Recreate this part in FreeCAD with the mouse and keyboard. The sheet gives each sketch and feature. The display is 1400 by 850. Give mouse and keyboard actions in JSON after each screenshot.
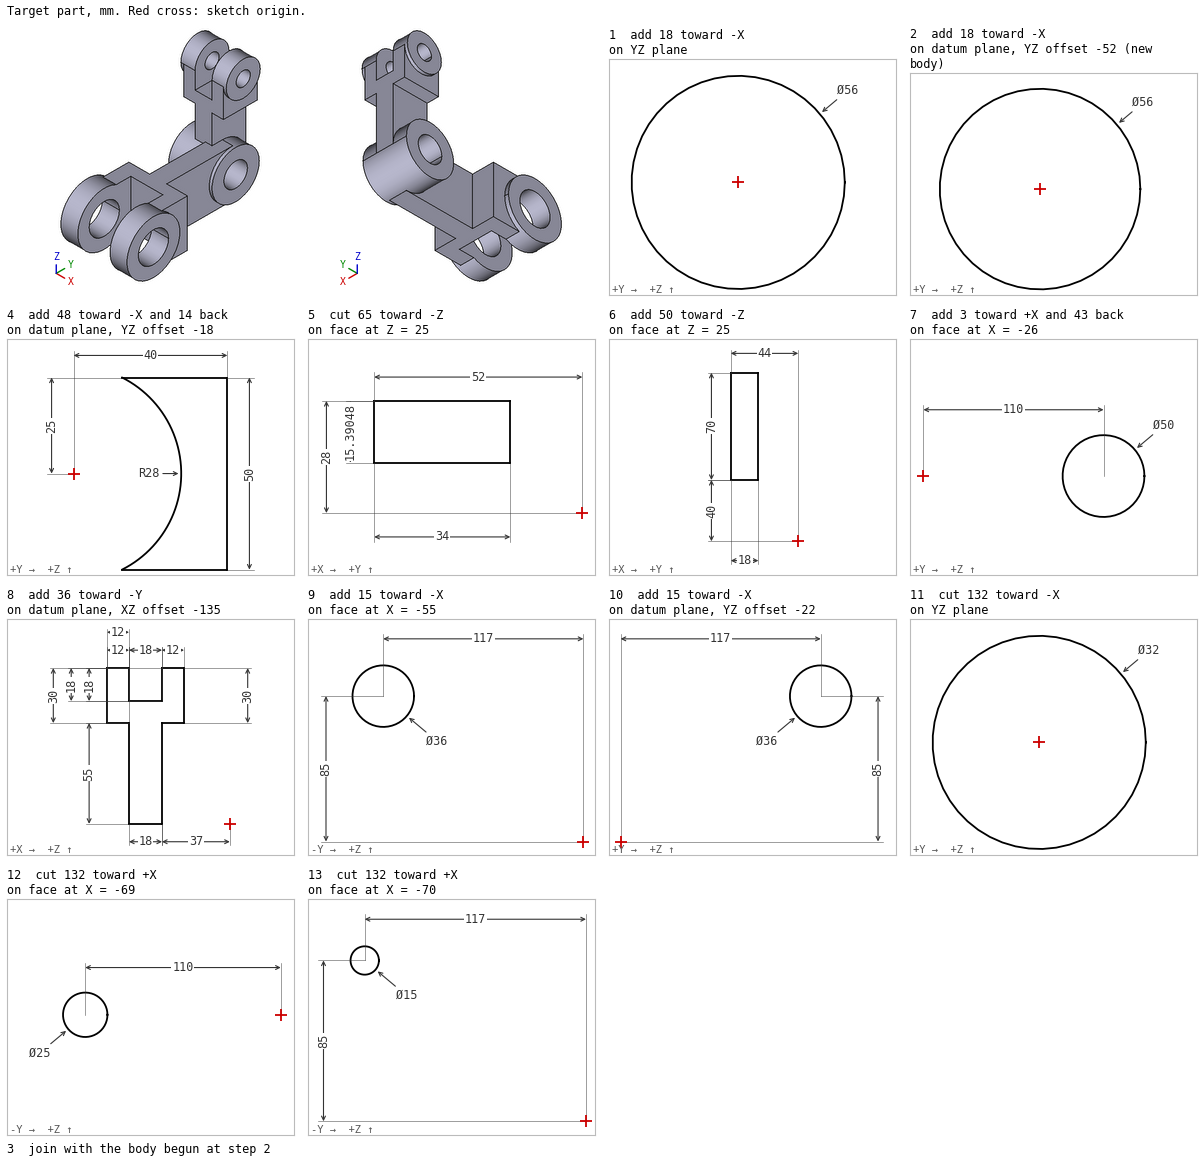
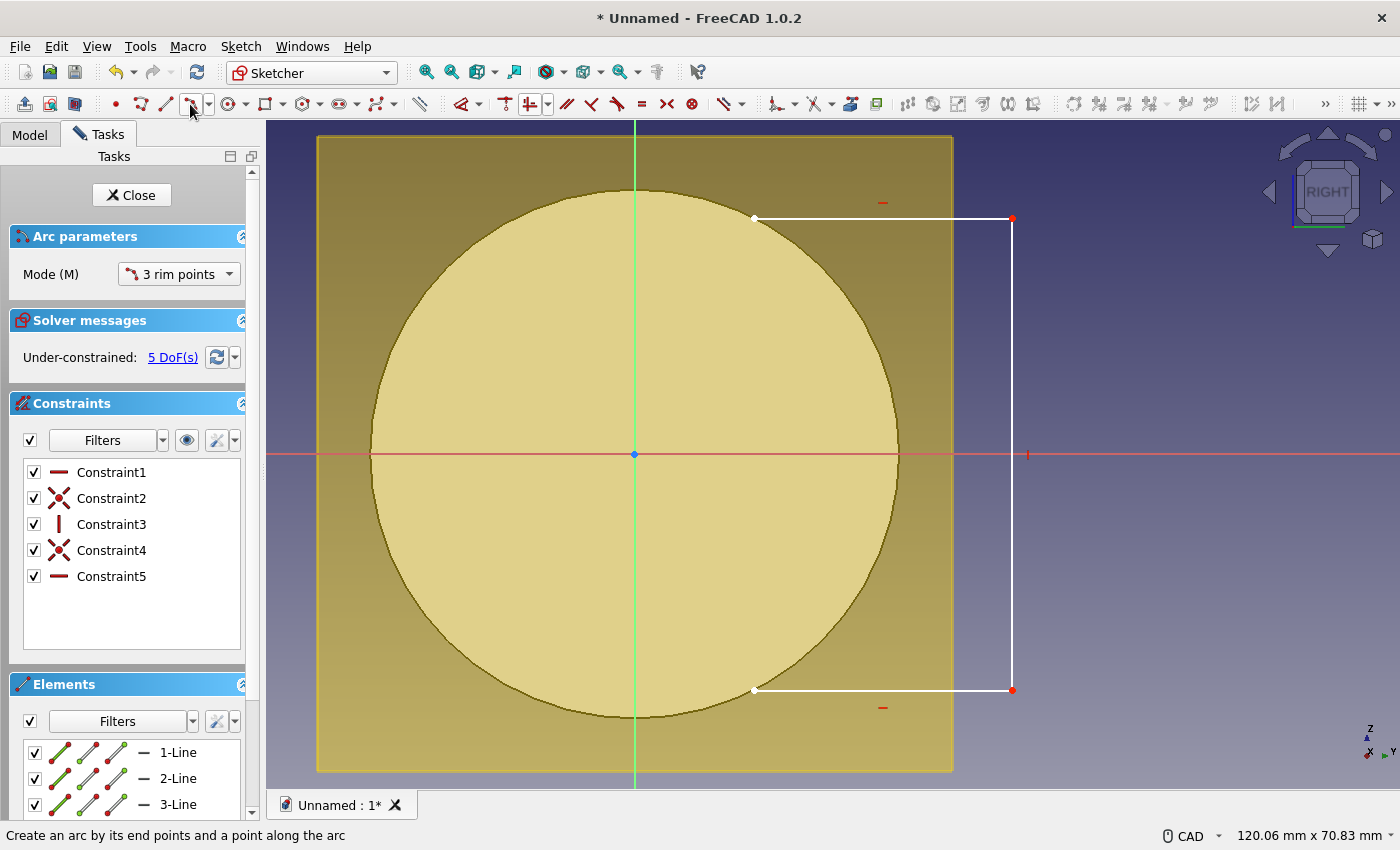
{"action": "left_click", "coordinate": [754, 691]}
{"action": "left_click", "coordinate": [754, 219]}
{"action": "left_click", "coordinate": [893, 512]}
{"action": "key", "text": "Escape"}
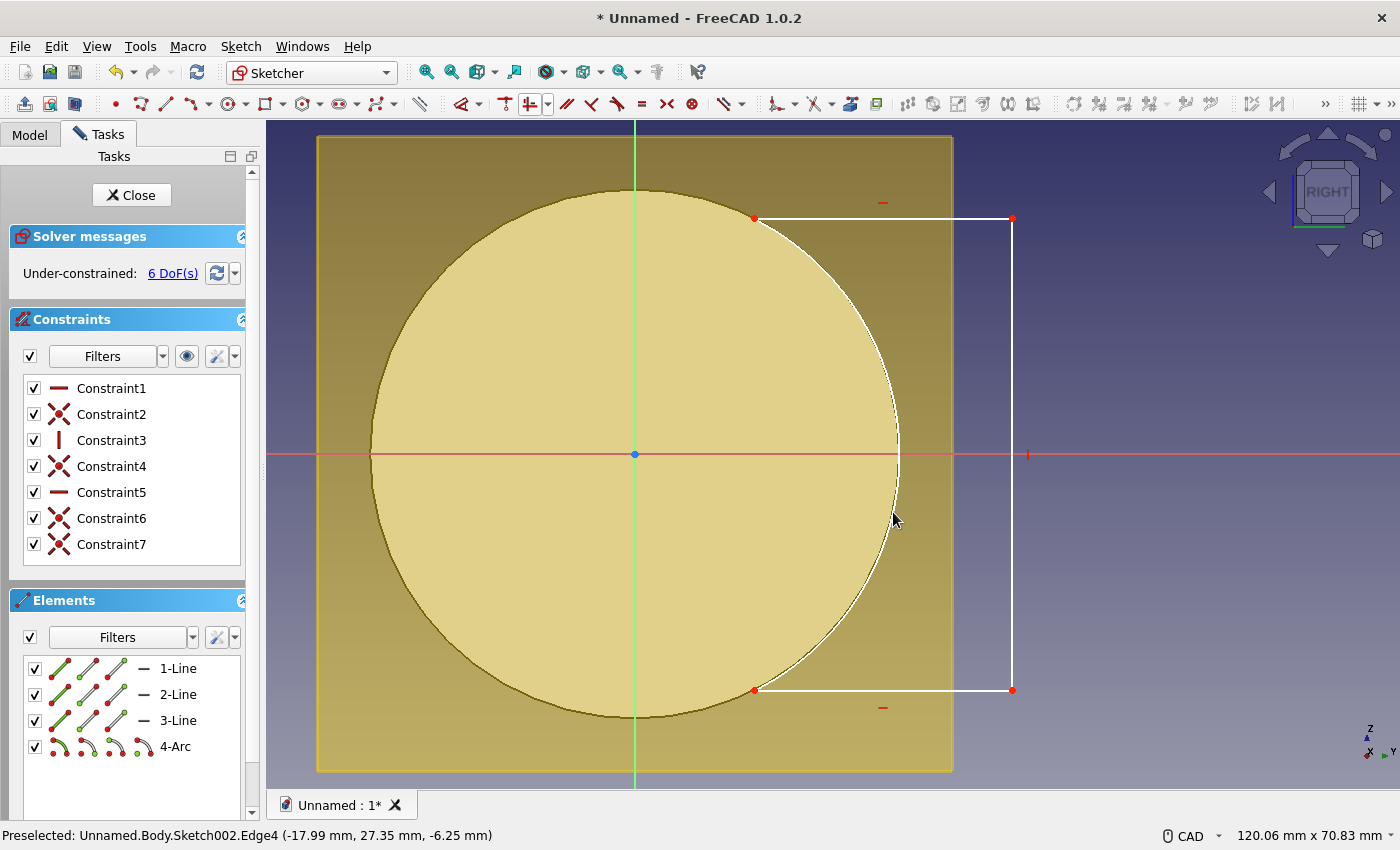
{"action": "left_click_drag", "start_coordinate": [625, 444], "coordinate": [645, 465]}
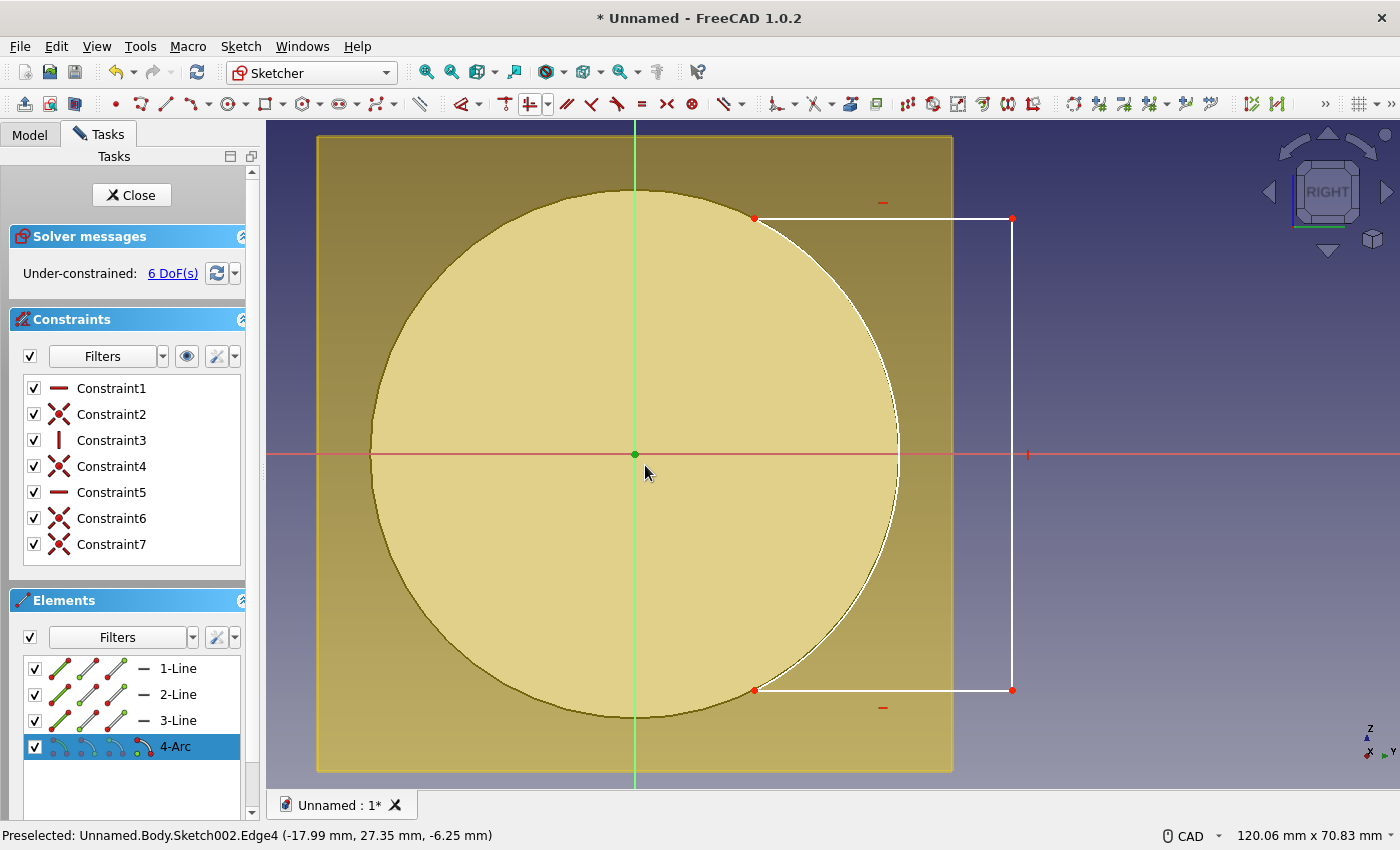
{"action": "key", "text": "c"}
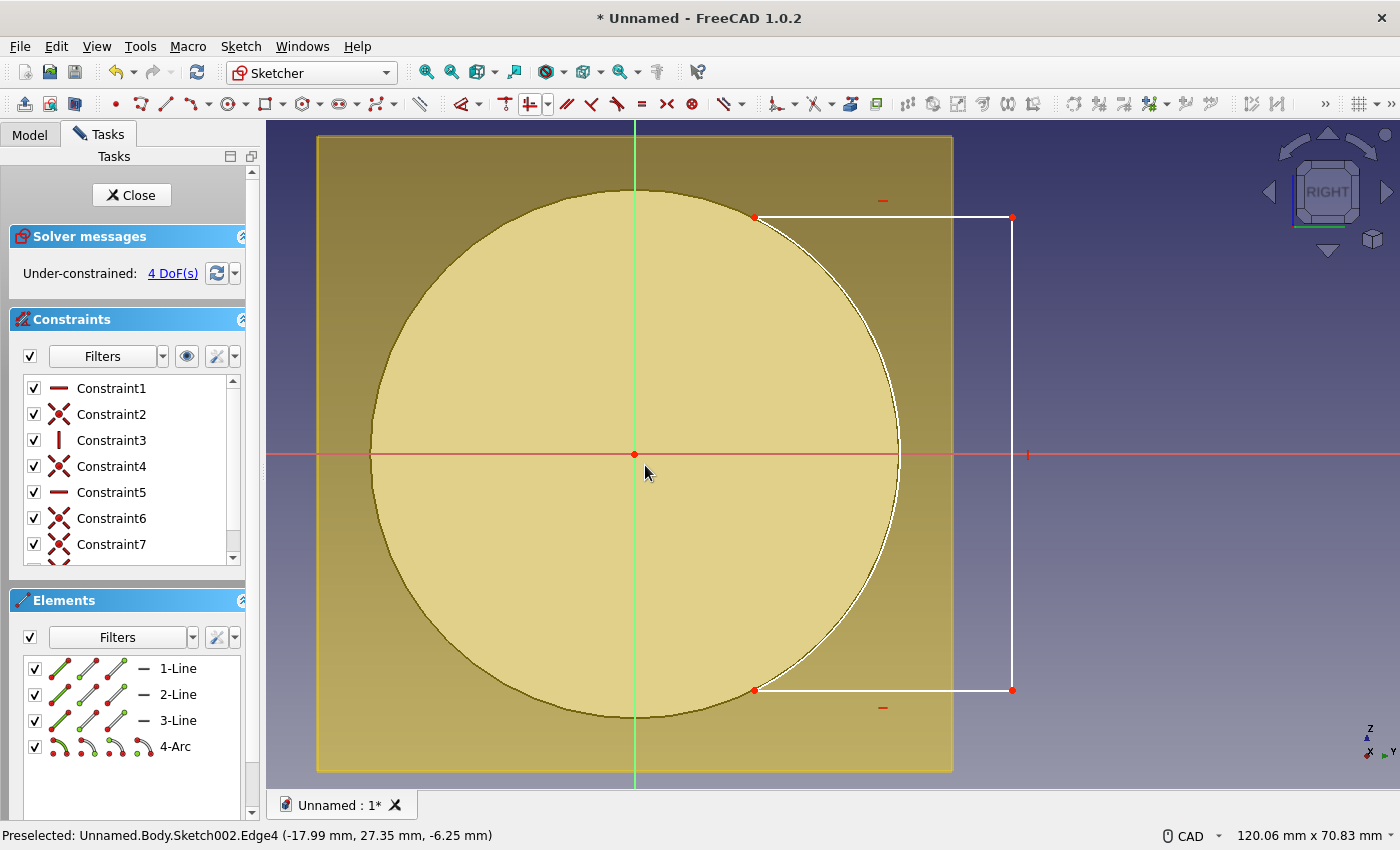
{"action": "left_click", "coordinate": [875, 567]}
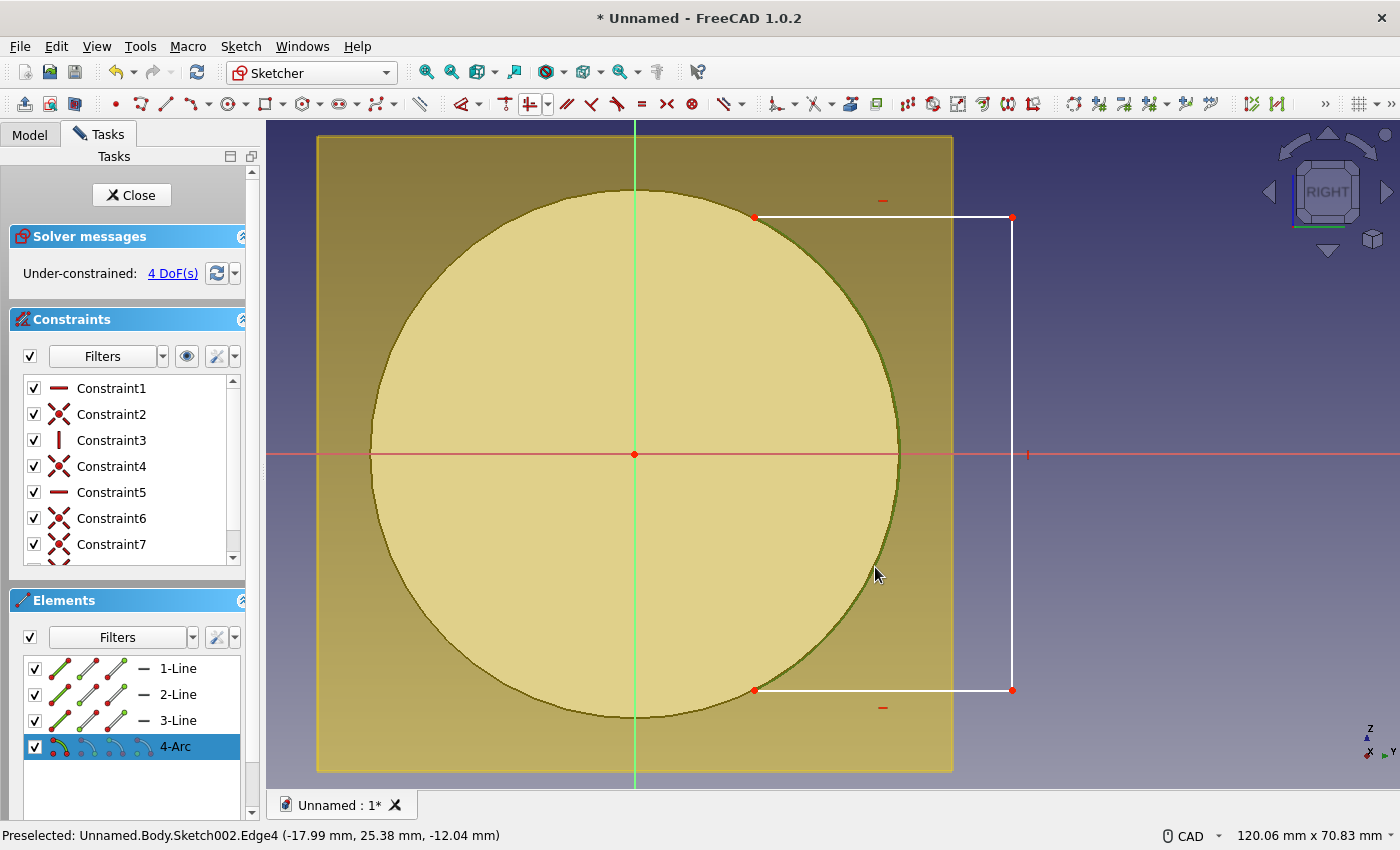
{"action": "key", "text": "k r"}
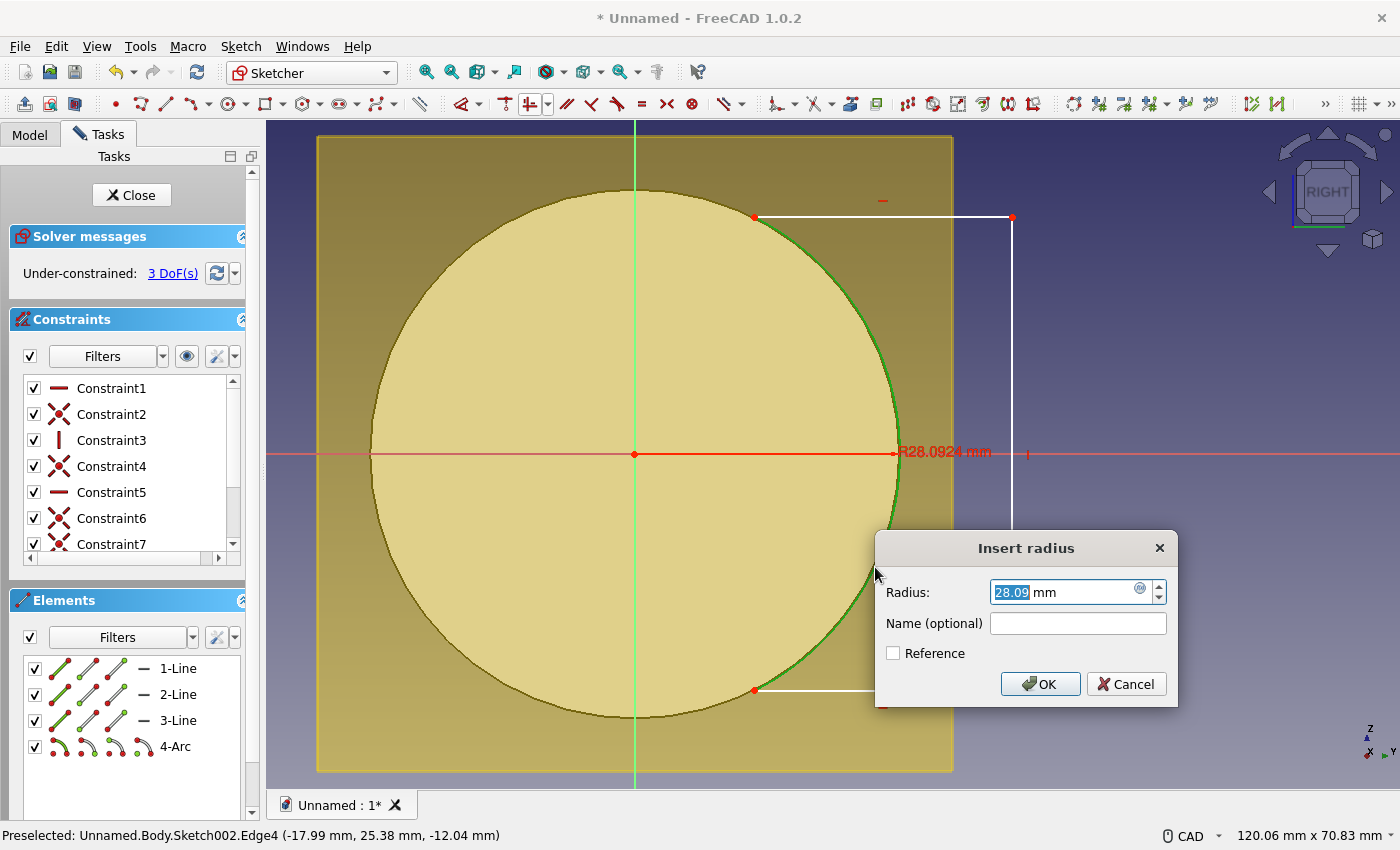
{"action": "type", "text": "28"}
{"action": "key", "text": "Return"}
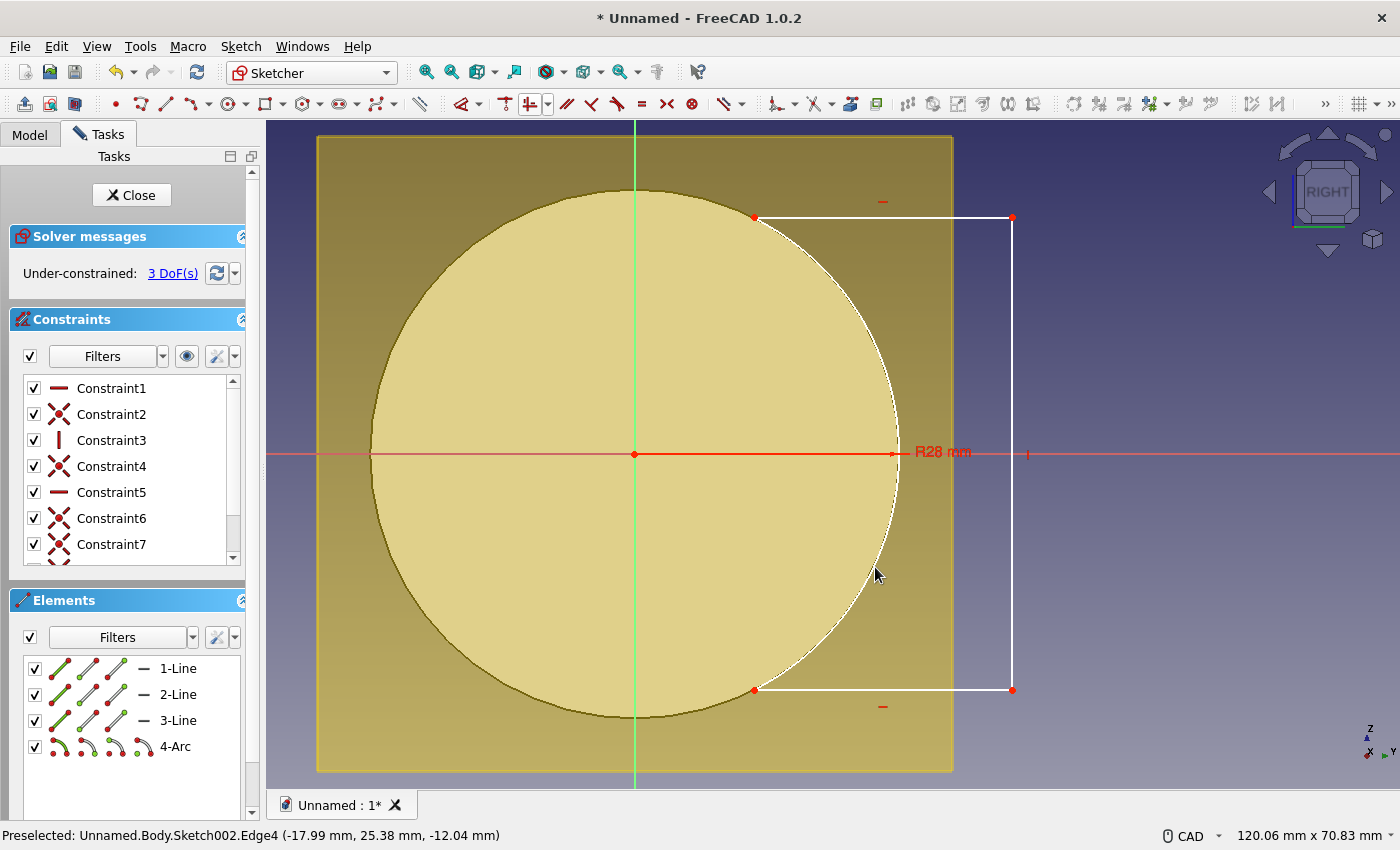
{"action": "left_click", "coordinate": [1012, 360]}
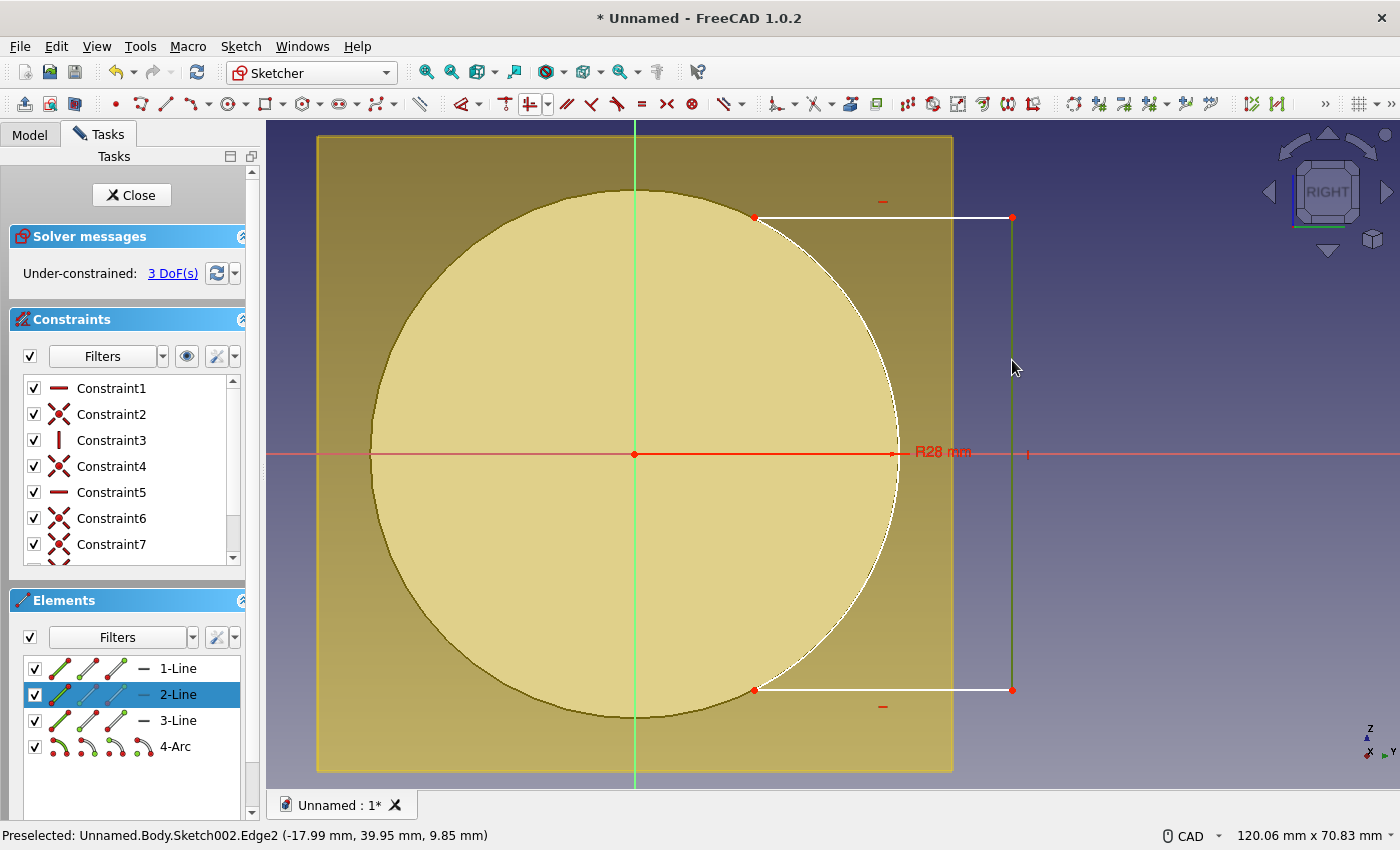
{"action": "key", "text": "i"}